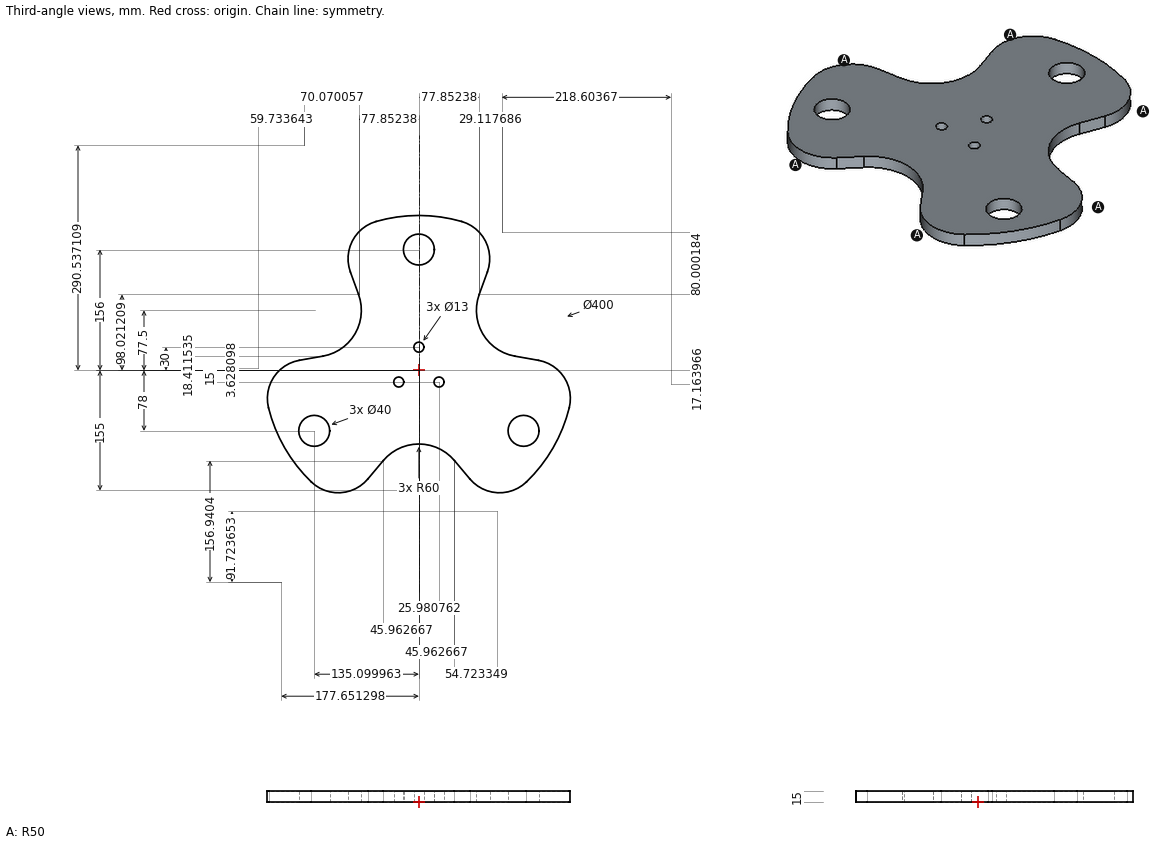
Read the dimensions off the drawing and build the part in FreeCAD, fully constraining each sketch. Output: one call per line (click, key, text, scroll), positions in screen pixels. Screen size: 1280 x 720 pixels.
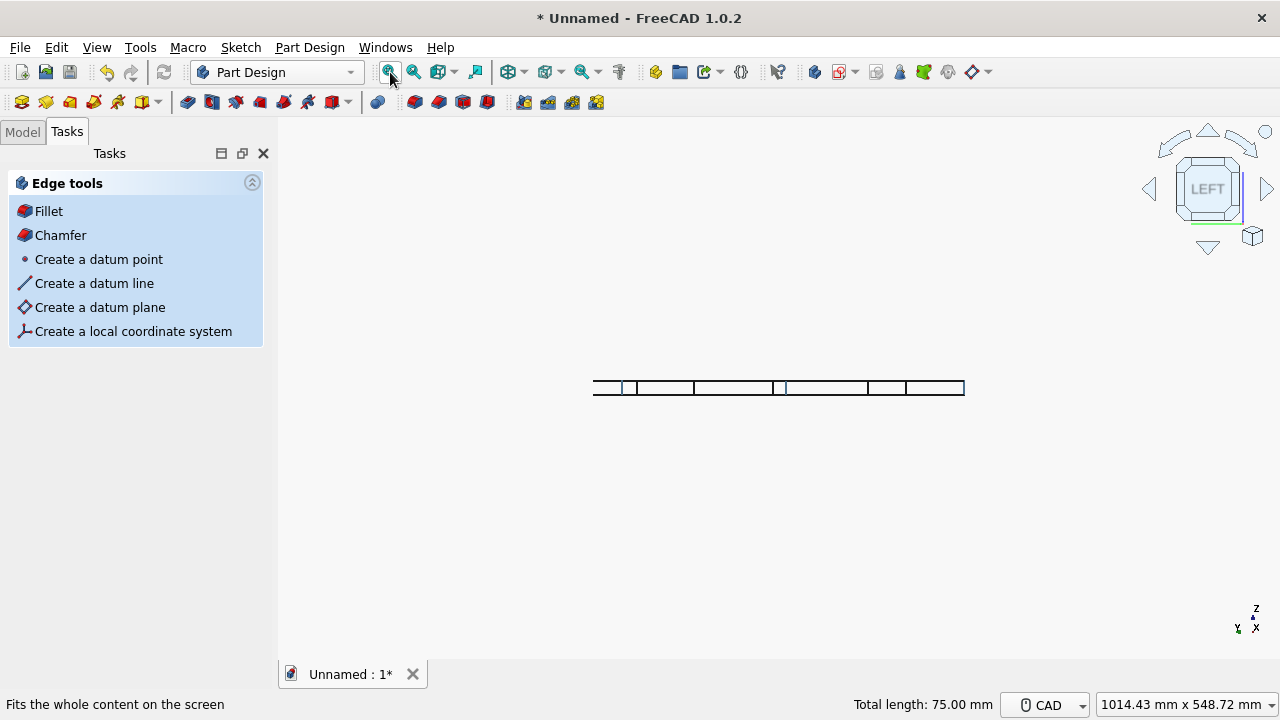
key(0)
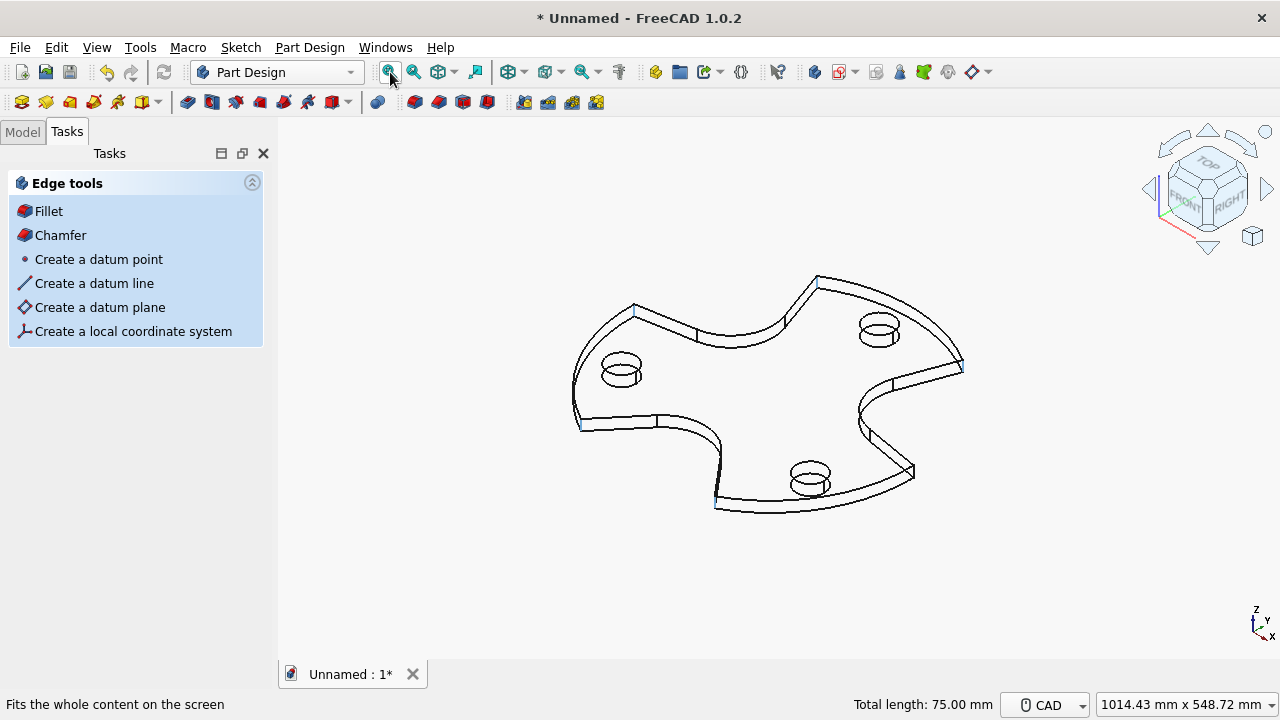
click(914, 472, ctrl)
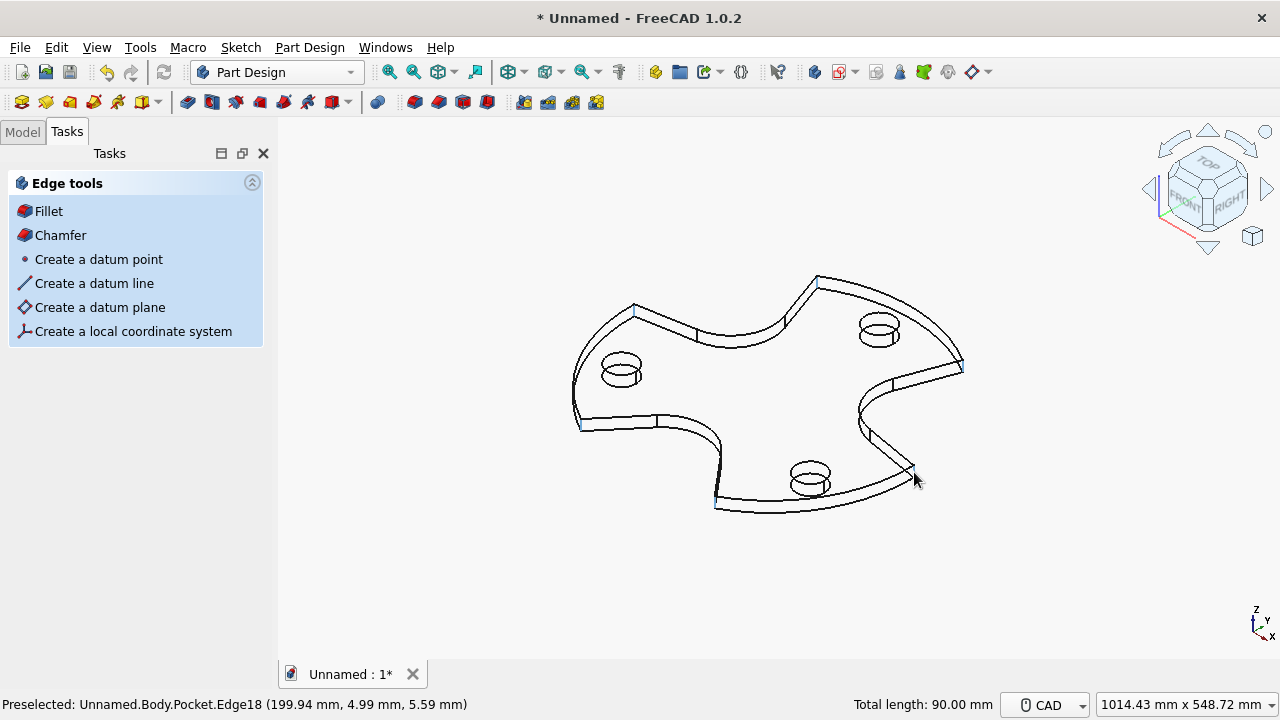
key(v)
key(1)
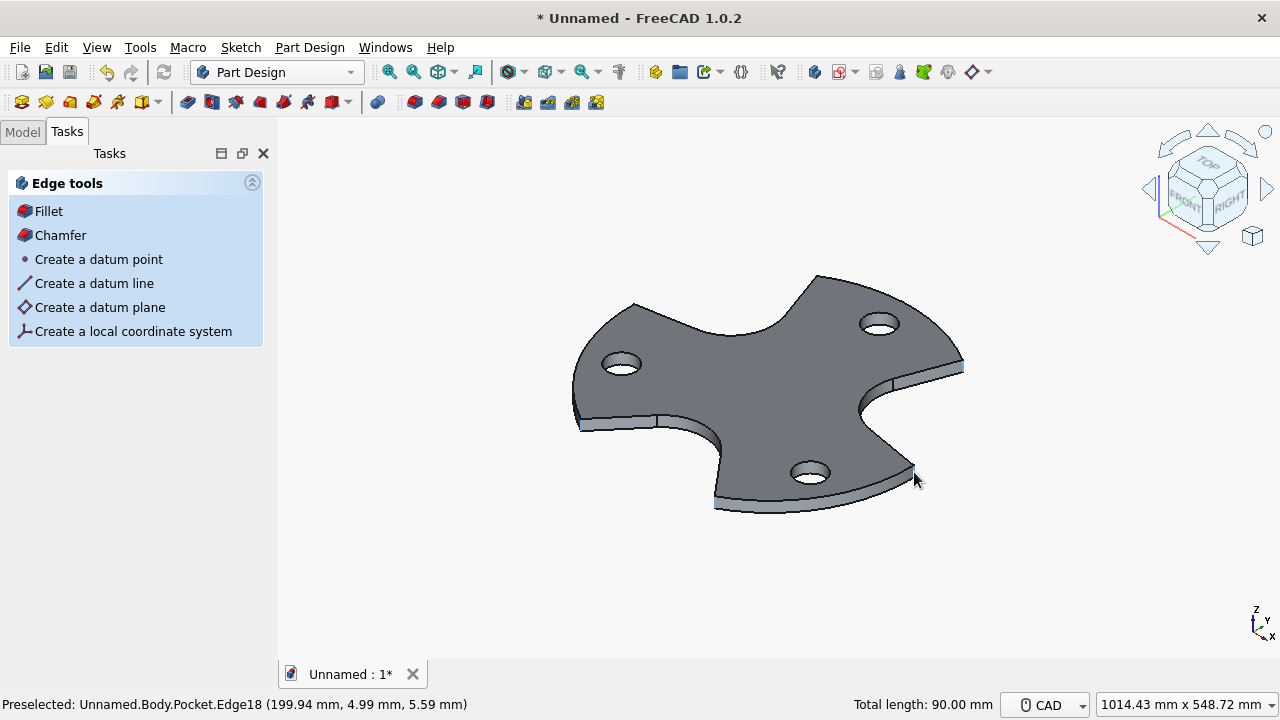
click(416, 102)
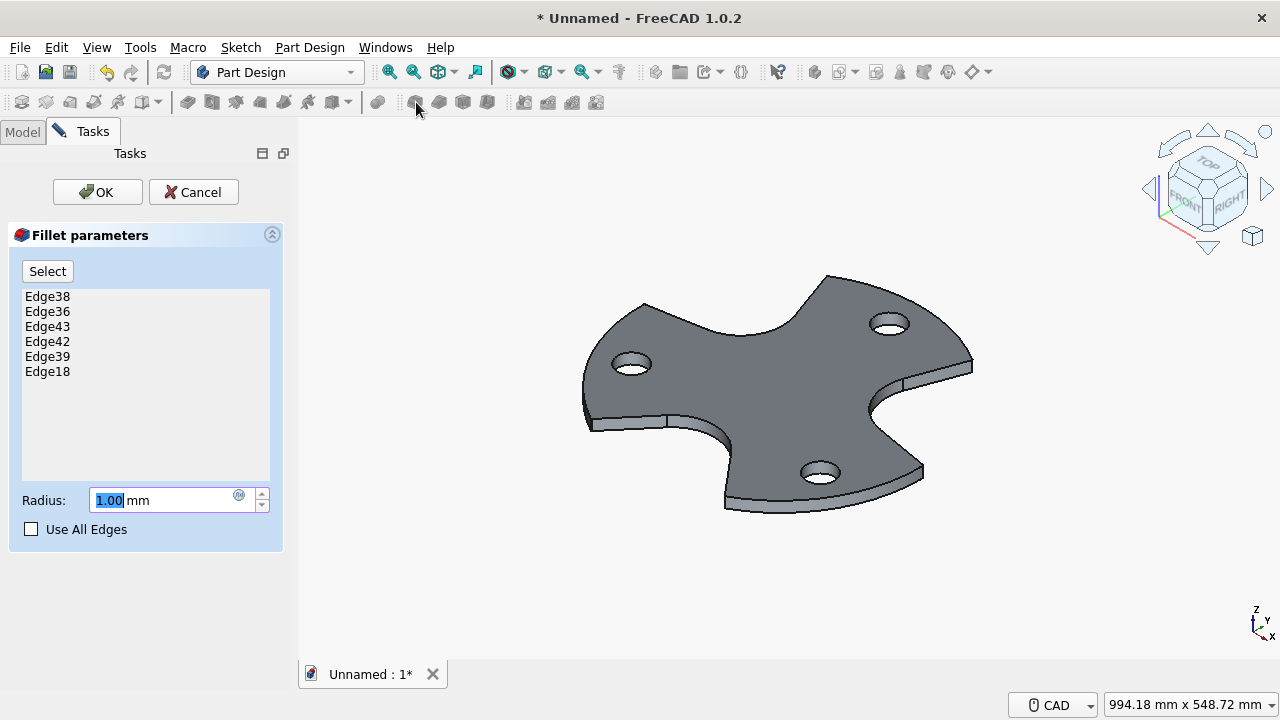
text(50)
key(Tab)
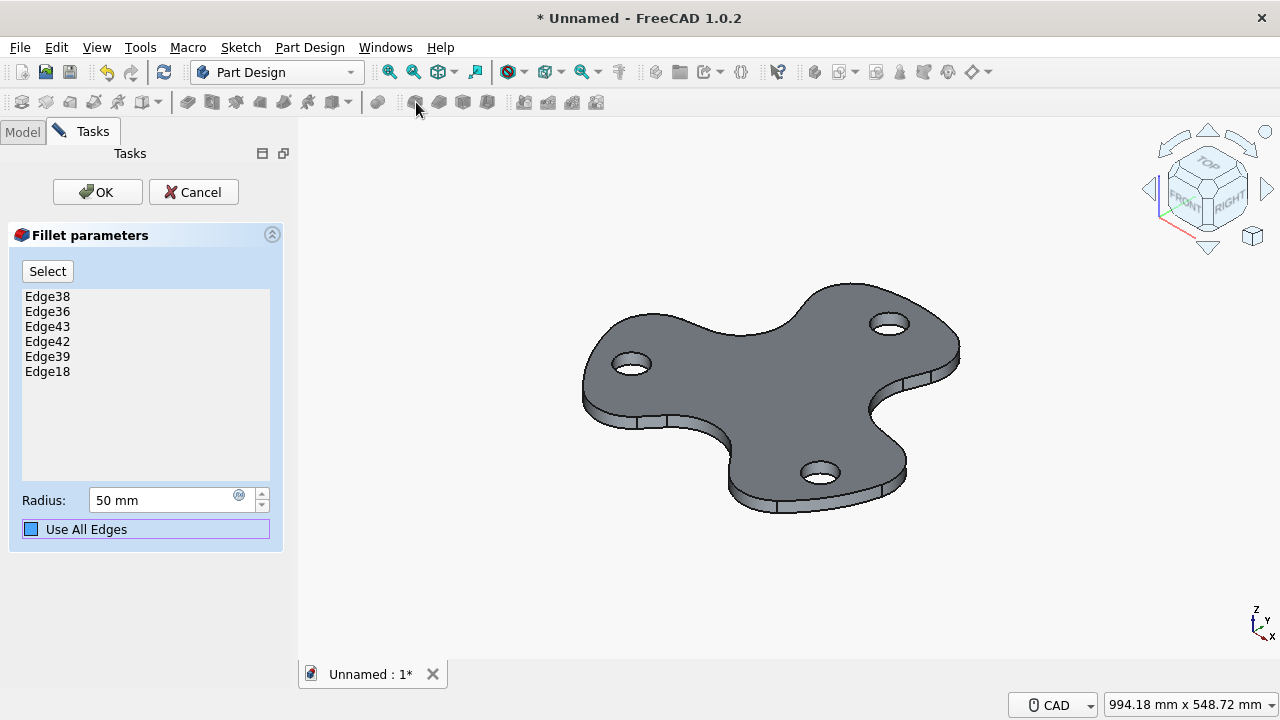
click(98, 192)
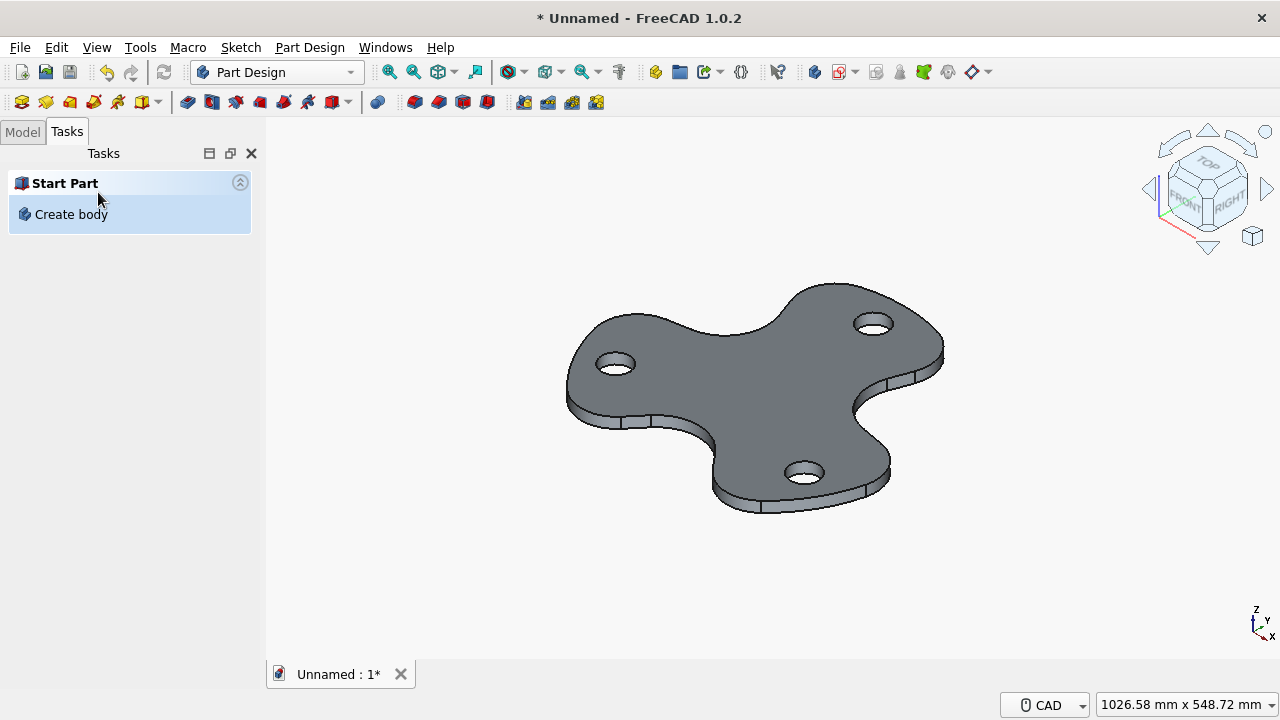
click(779, 377)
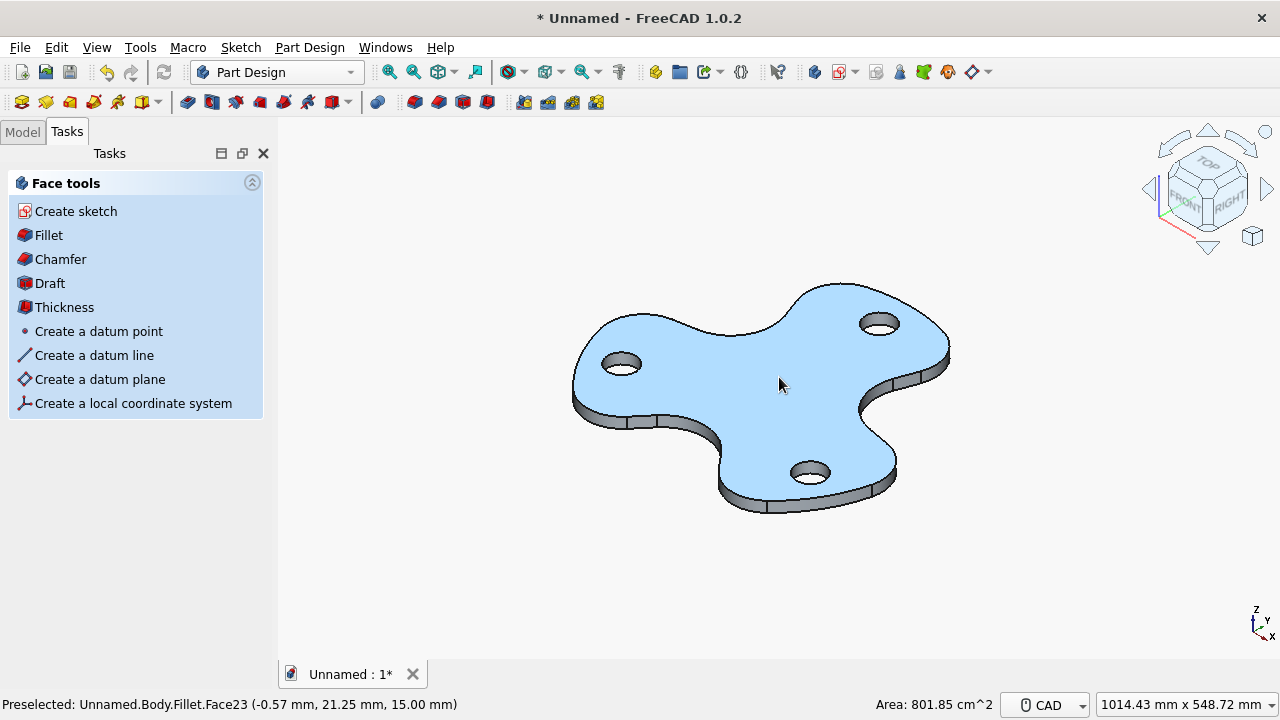
click(840, 72)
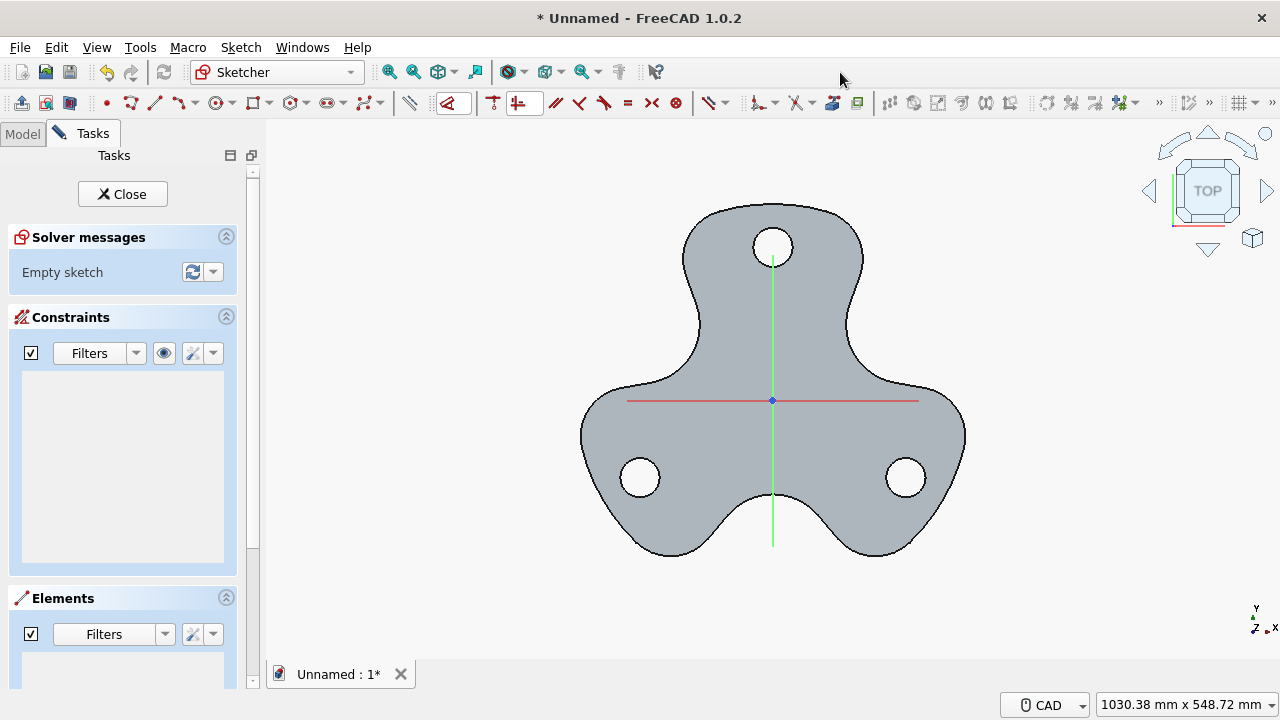
scroll(787, 394, up, 9)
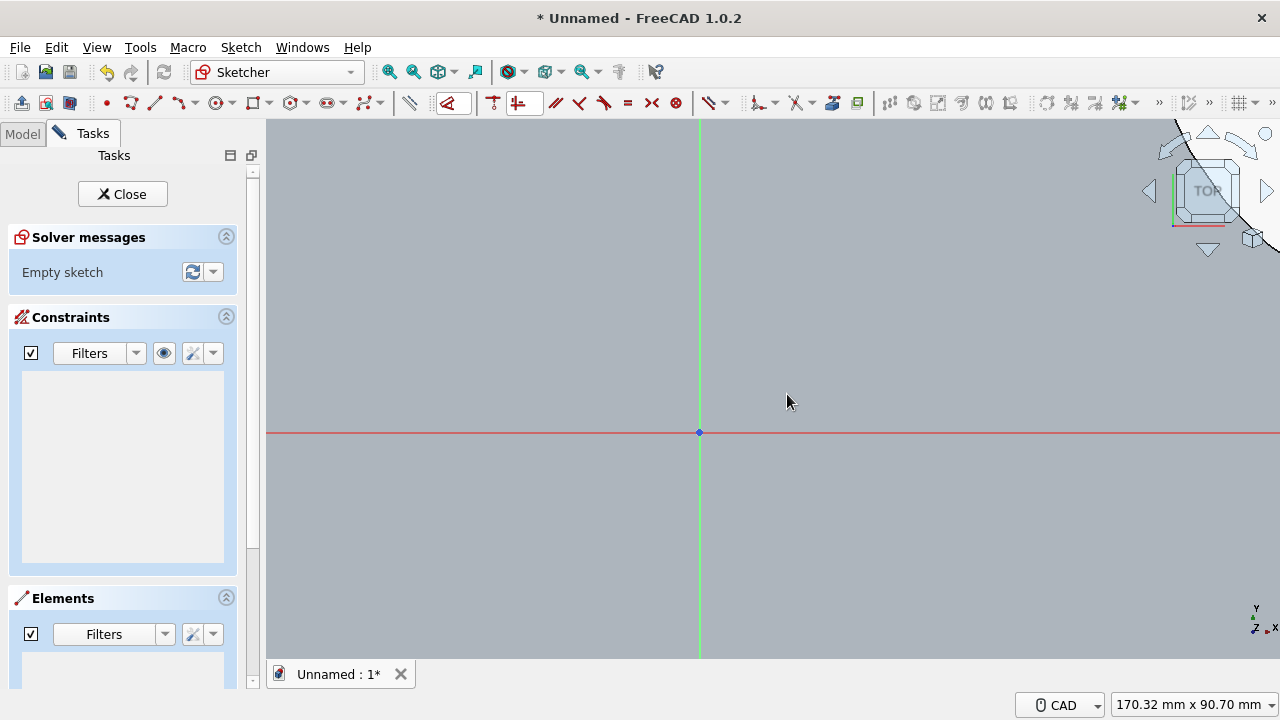
click(216, 104)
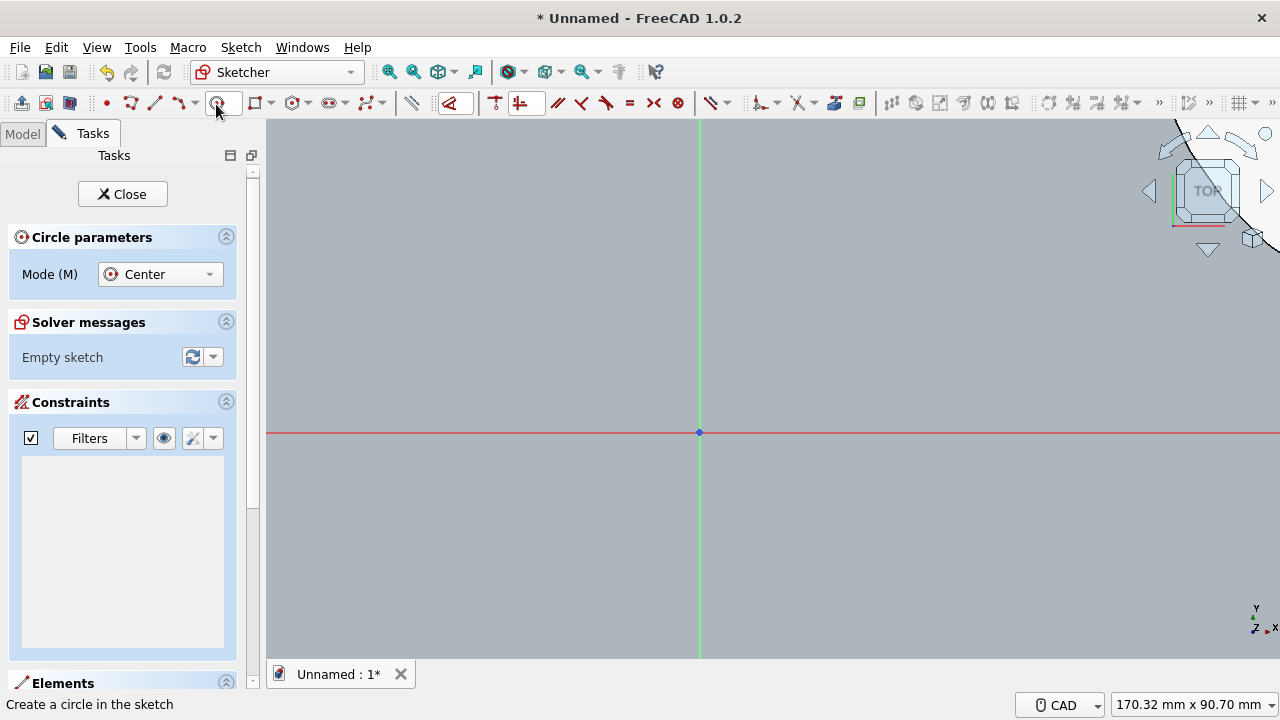
click(700, 254)
move(727, 227)